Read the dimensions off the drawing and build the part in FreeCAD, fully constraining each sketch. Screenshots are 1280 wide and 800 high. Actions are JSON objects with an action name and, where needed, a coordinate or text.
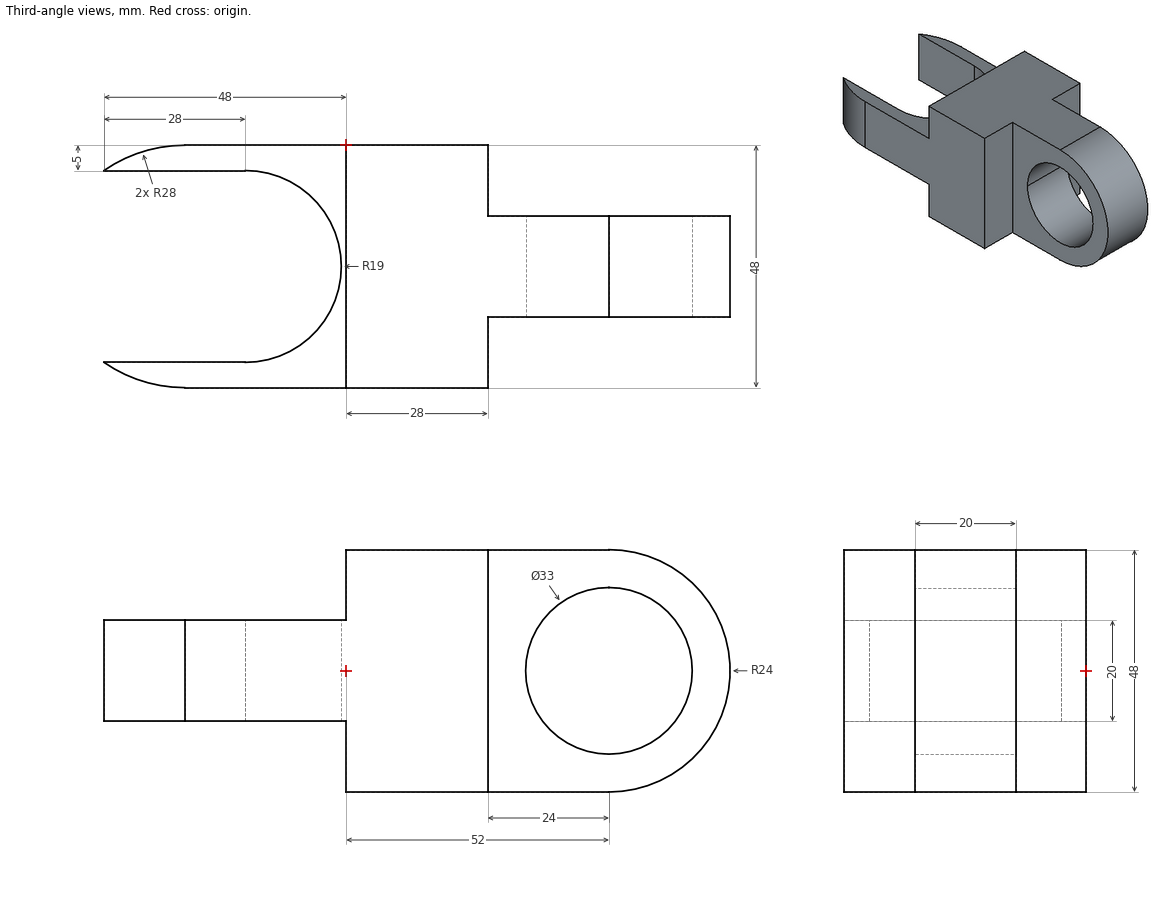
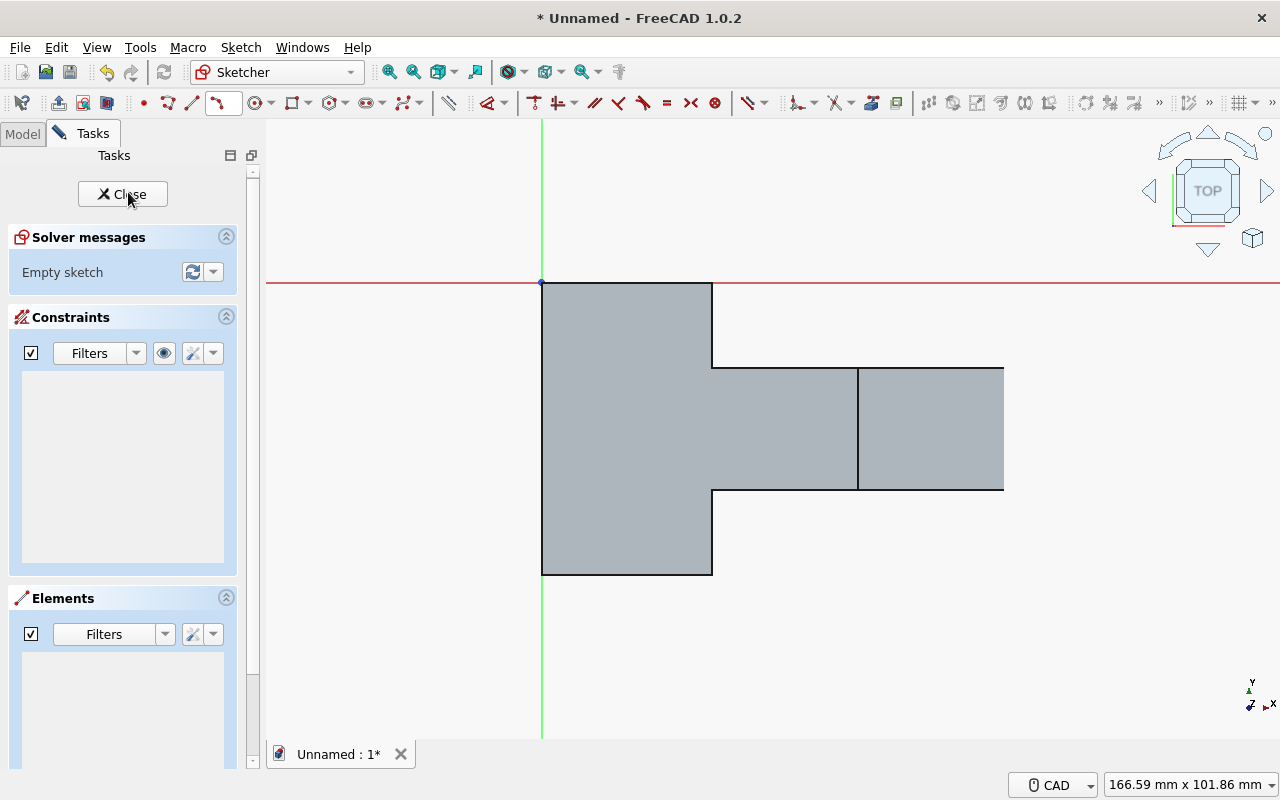
{"action": "left_click", "coordinate": [108, 104]}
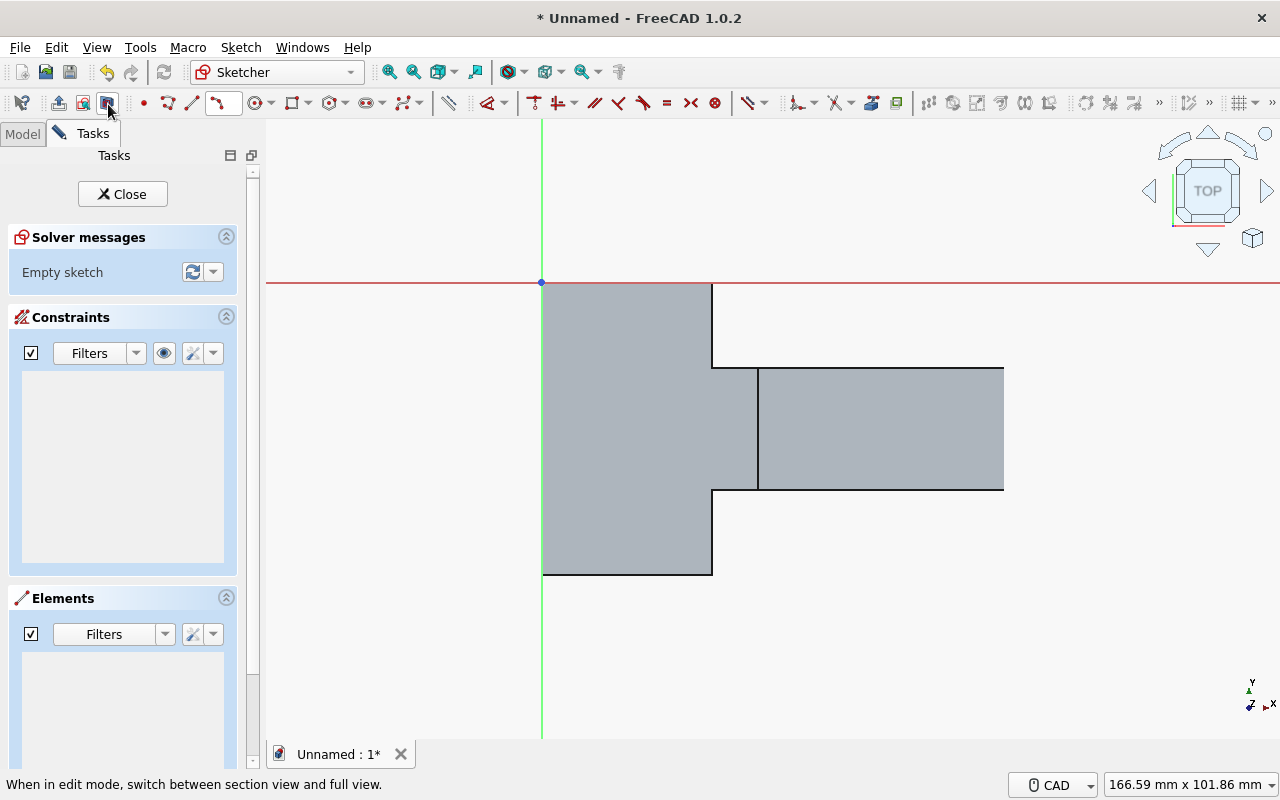
{"action": "scroll", "coordinate": [1115, 429], "scroll_direction": "down", "scroll_amount": 1}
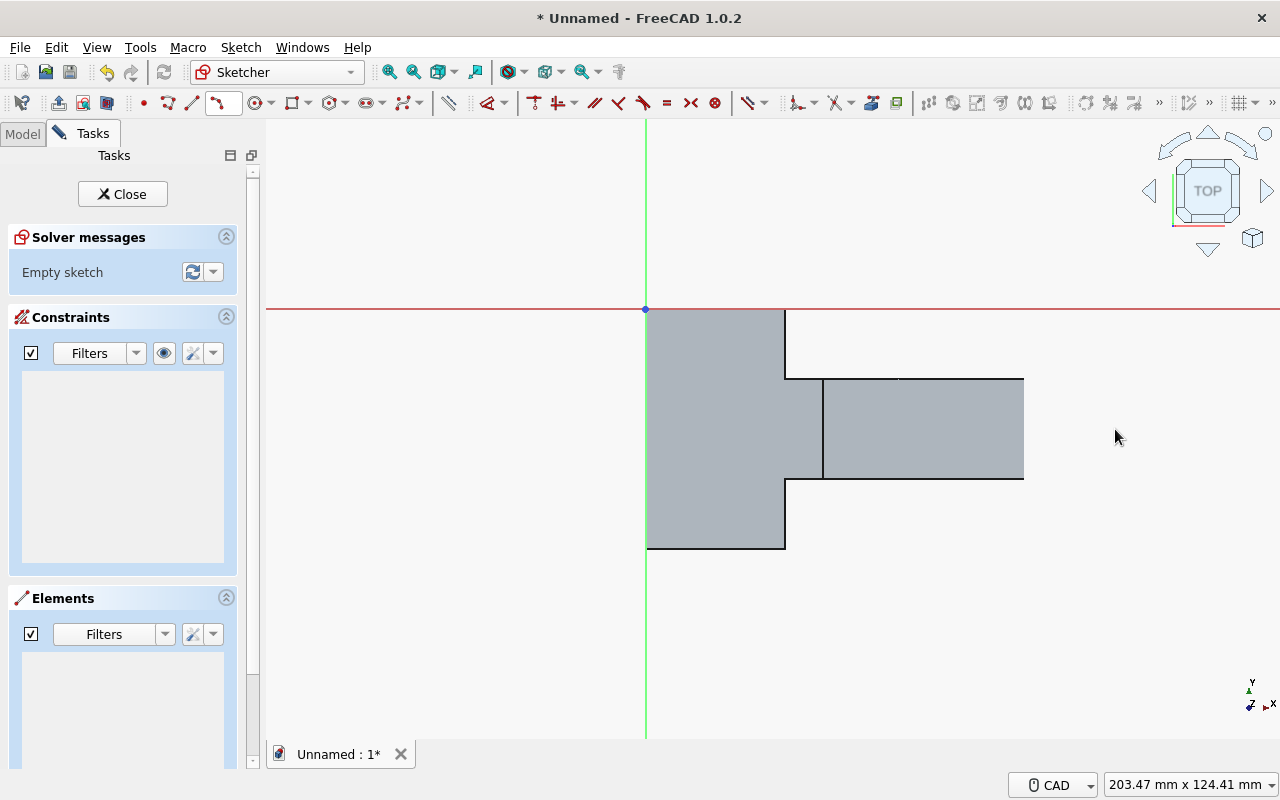
{"action": "scroll", "coordinate": [310, 429], "scroll_direction": "up", "scroll_amount": 3}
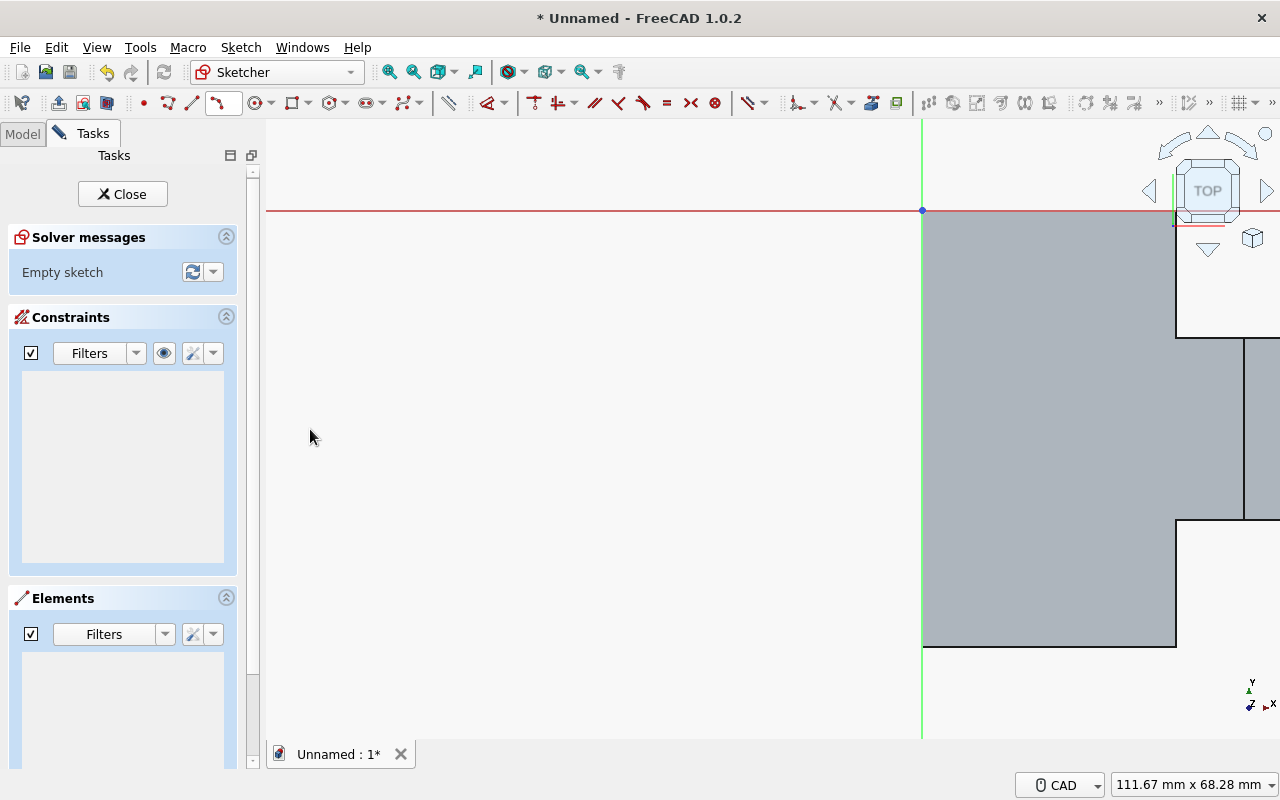
{"action": "key", "text": "g l"}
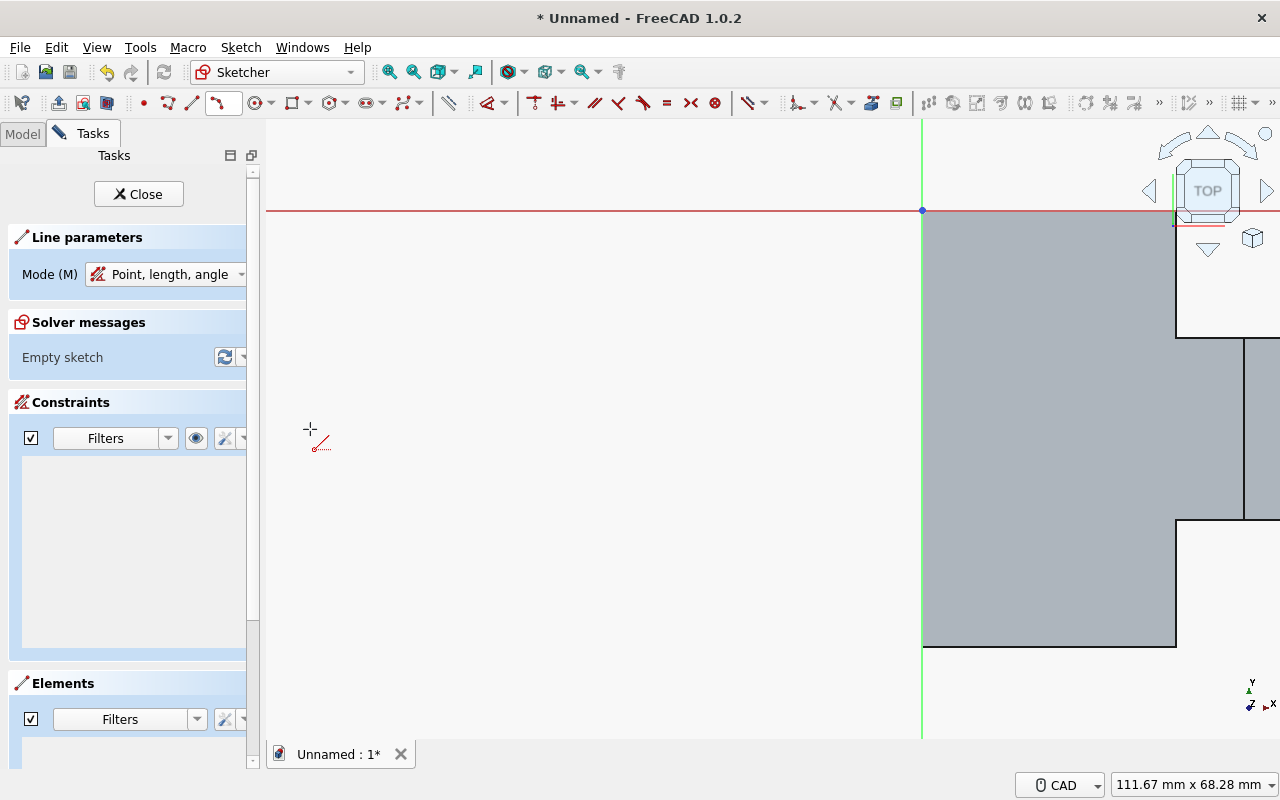
{"action": "left_click", "coordinate": [486, 256]}
{"action": "left_click", "coordinate": [740, 256]}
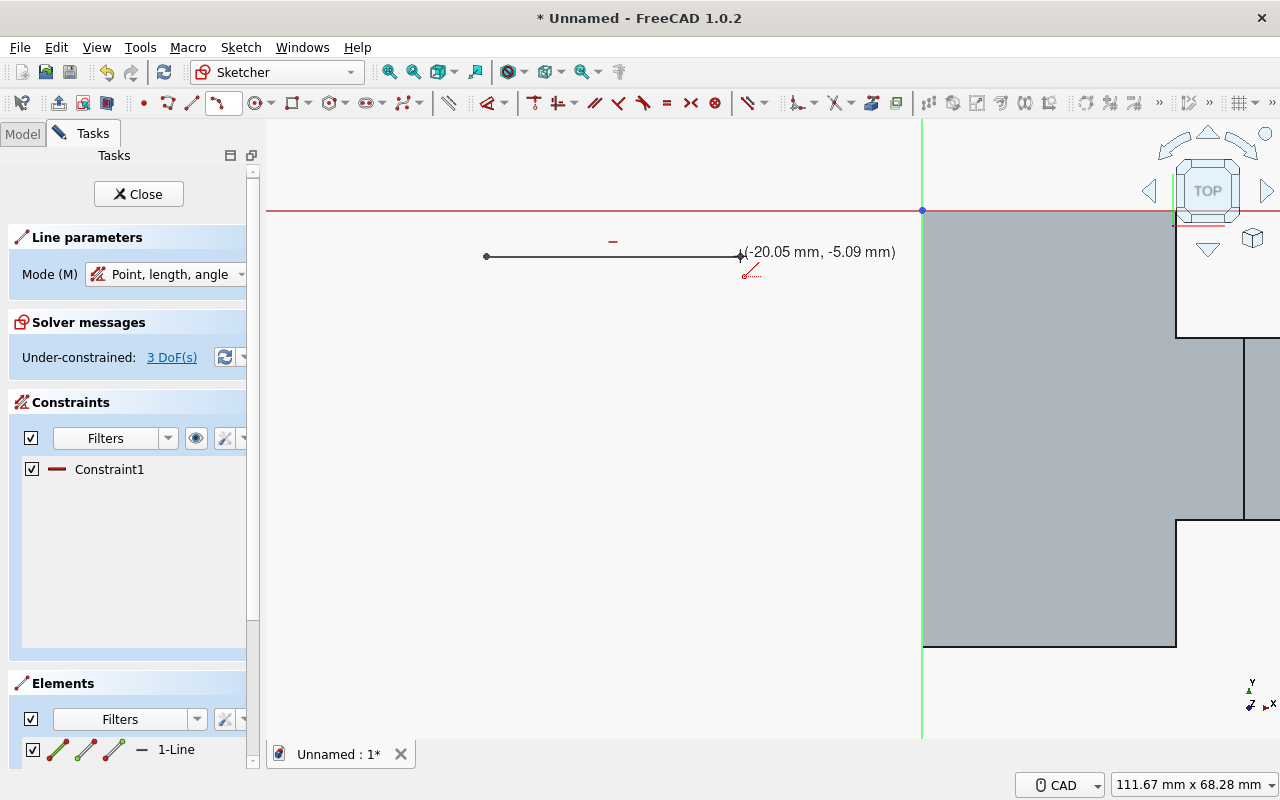
{"action": "left_click", "coordinate": [740, 601]}
{"action": "left_click", "coordinate": [486, 601]}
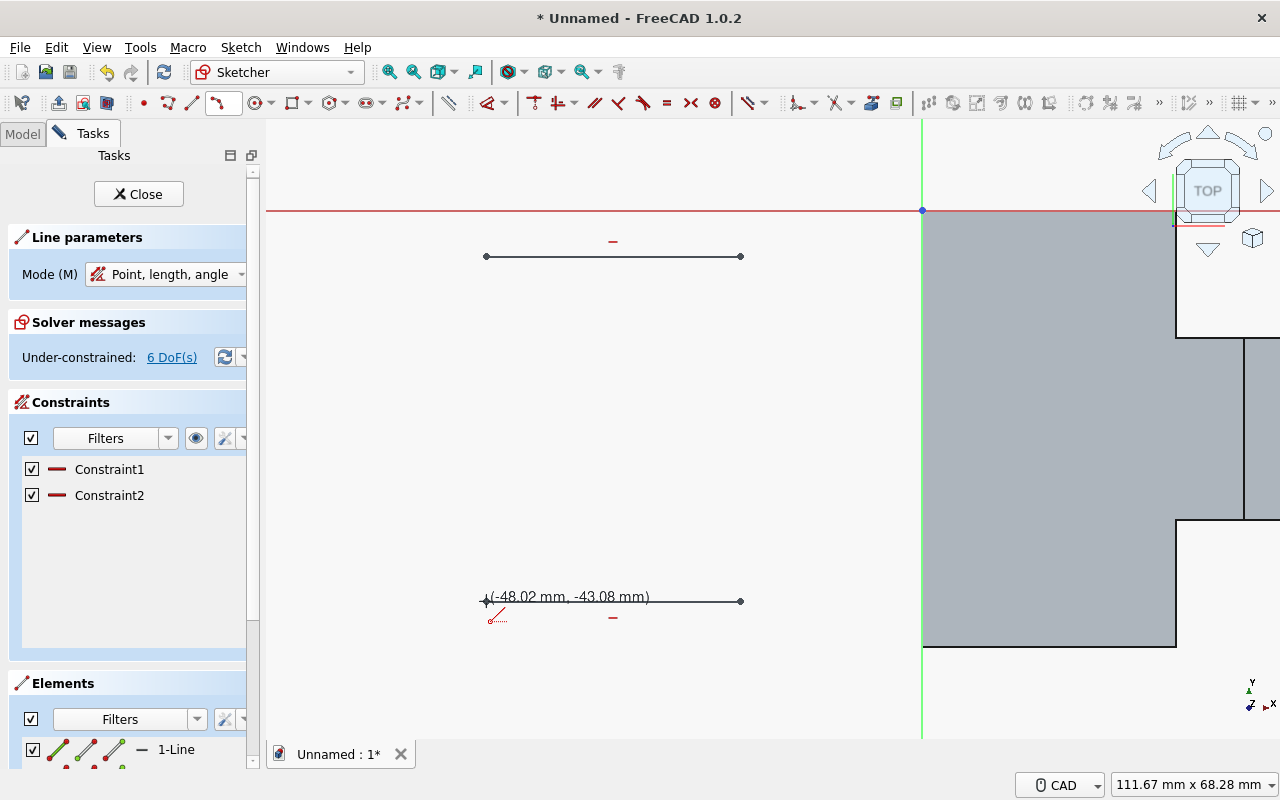
{"action": "left_click", "coordinate": [168, 104]}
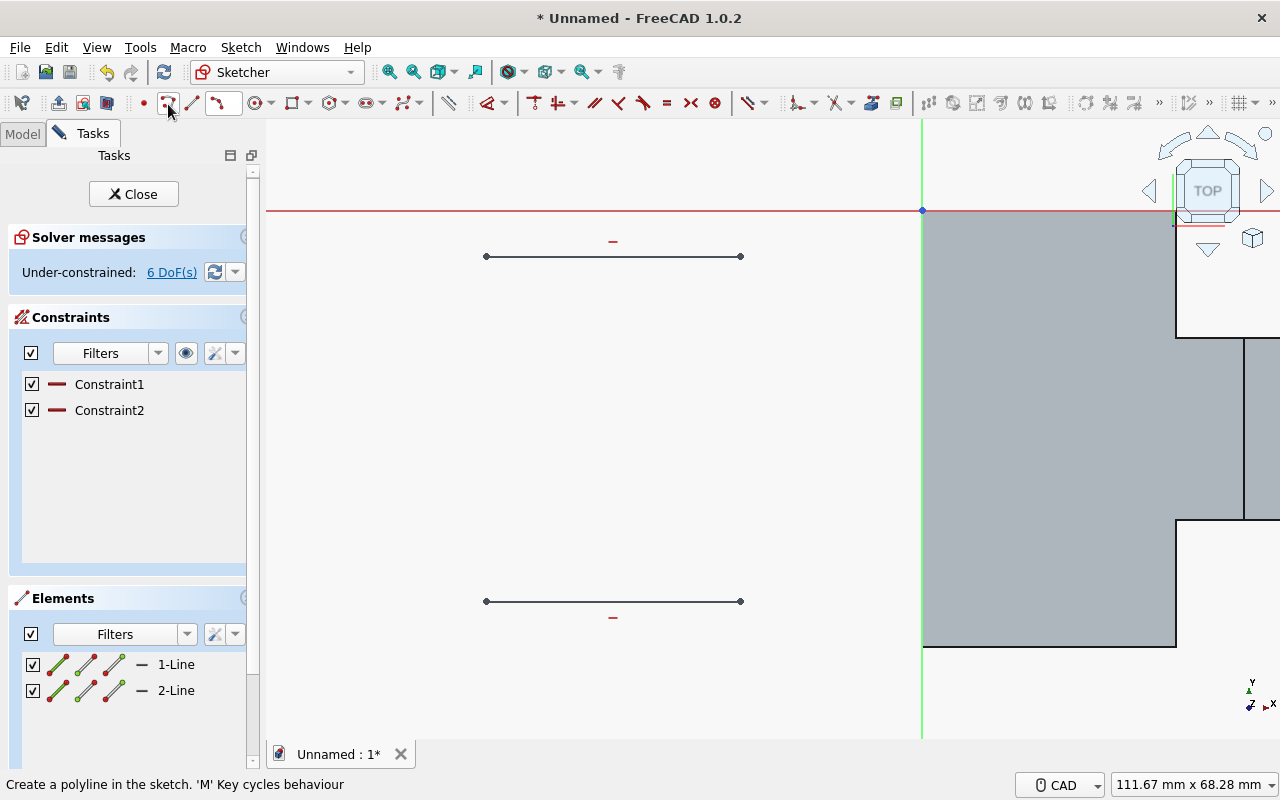
{"action": "left_click", "coordinate": [631, 647]}
{"action": "left_click", "coordinate": [922, 647]}
{"action": "left_click", "coordinate": [922, 211]}
{"action": "left_click", "coordinate": [631, 220]}
{"action": "right_click", "coordinate": [631, 220]}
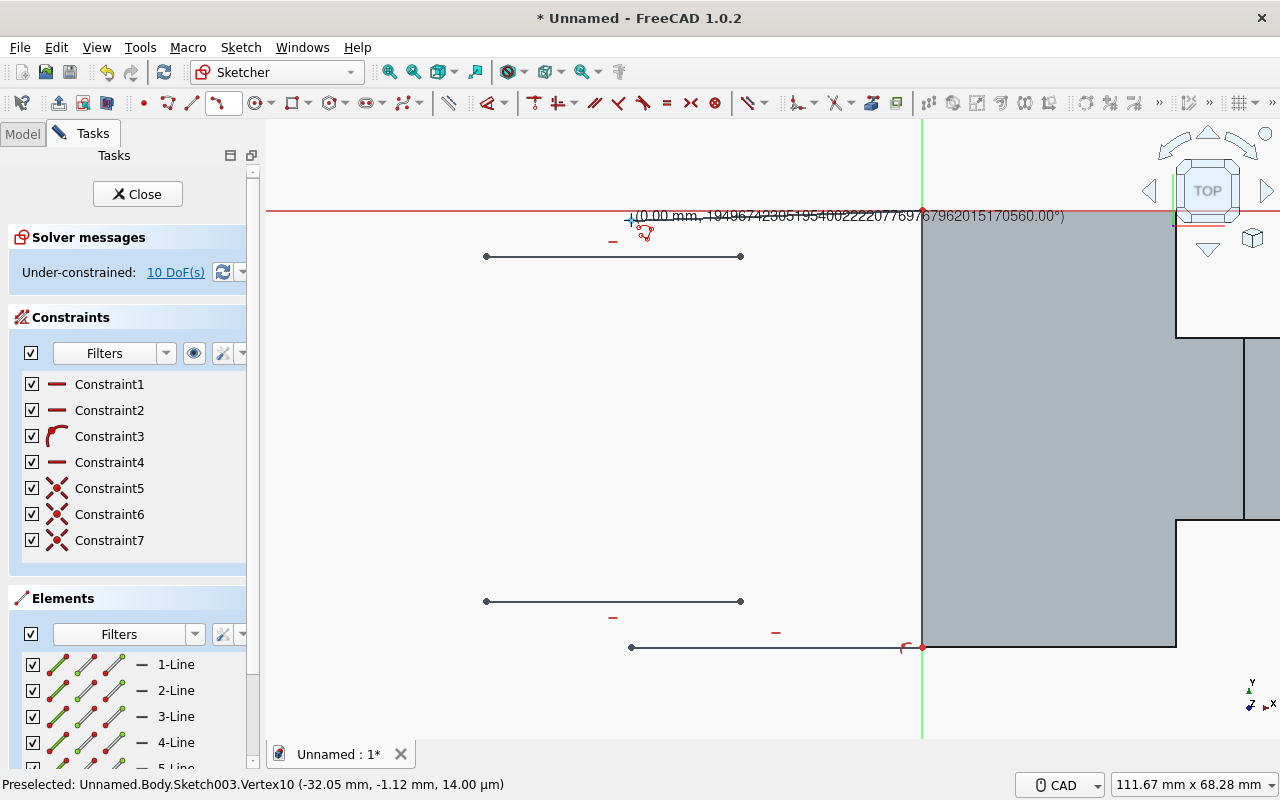
{"action": "left_click", "coordinate": [218, 104]}